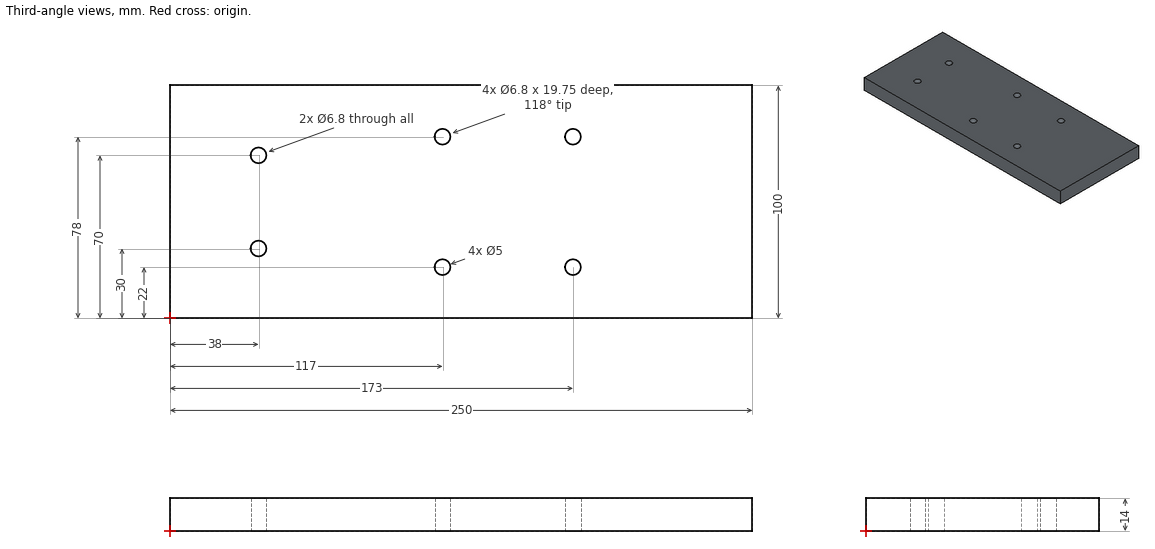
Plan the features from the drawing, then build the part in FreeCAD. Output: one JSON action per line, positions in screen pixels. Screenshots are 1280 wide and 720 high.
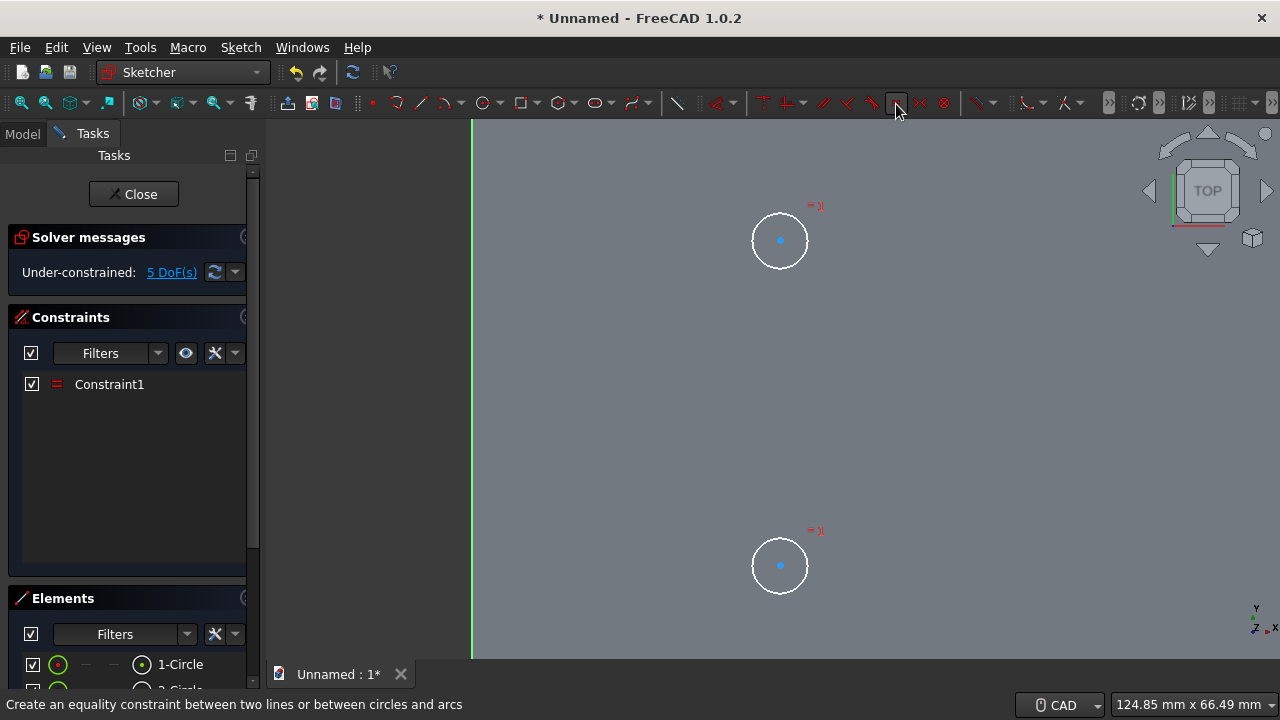
{"action": "left_click", "coordinate": [716, 104]}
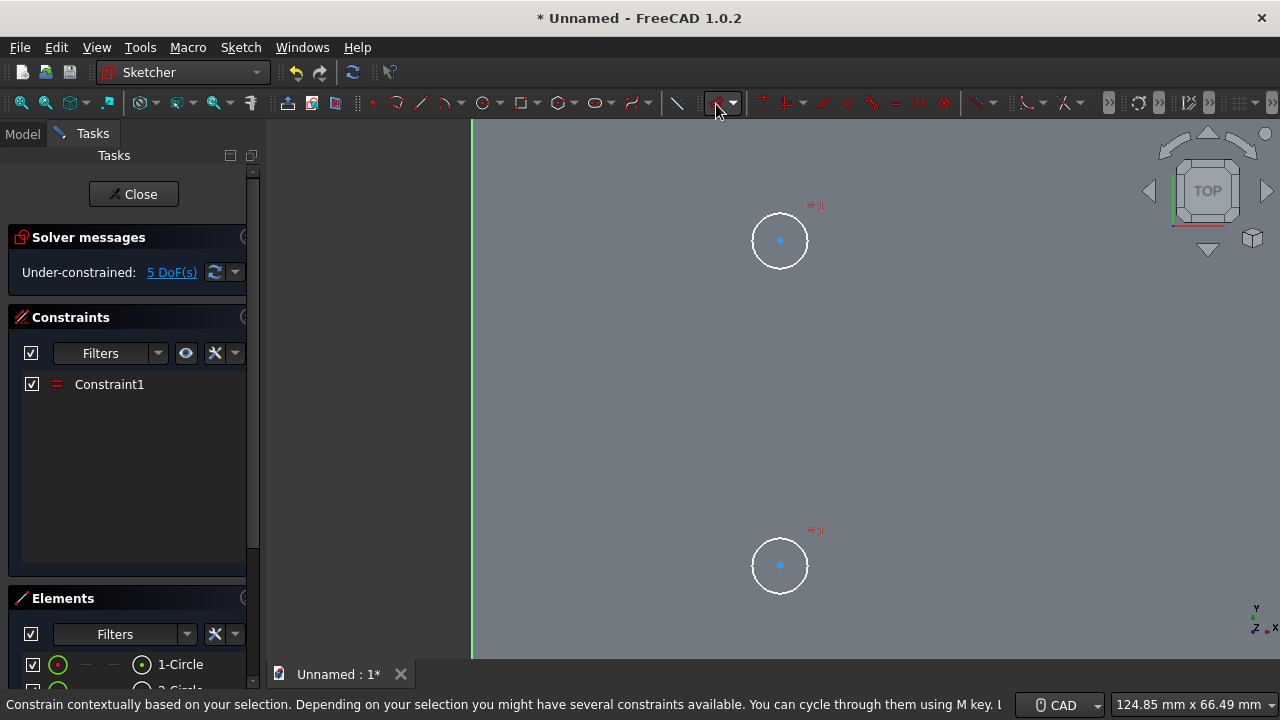
{"action": "left_click", "coordinate": [799, 221]}
{"action": "left_click", "coordinate": [821, 198]}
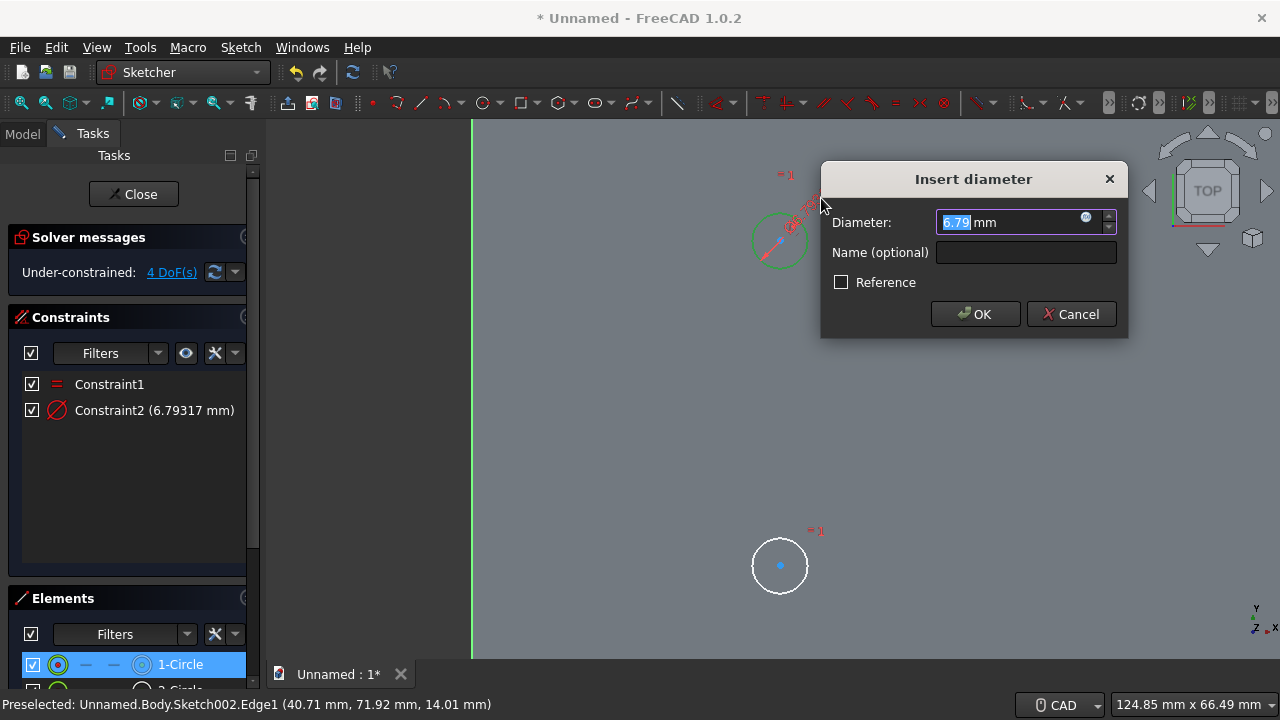
{"action": "type", "text": "6.8"}
{"action": "key", "text": "Return"}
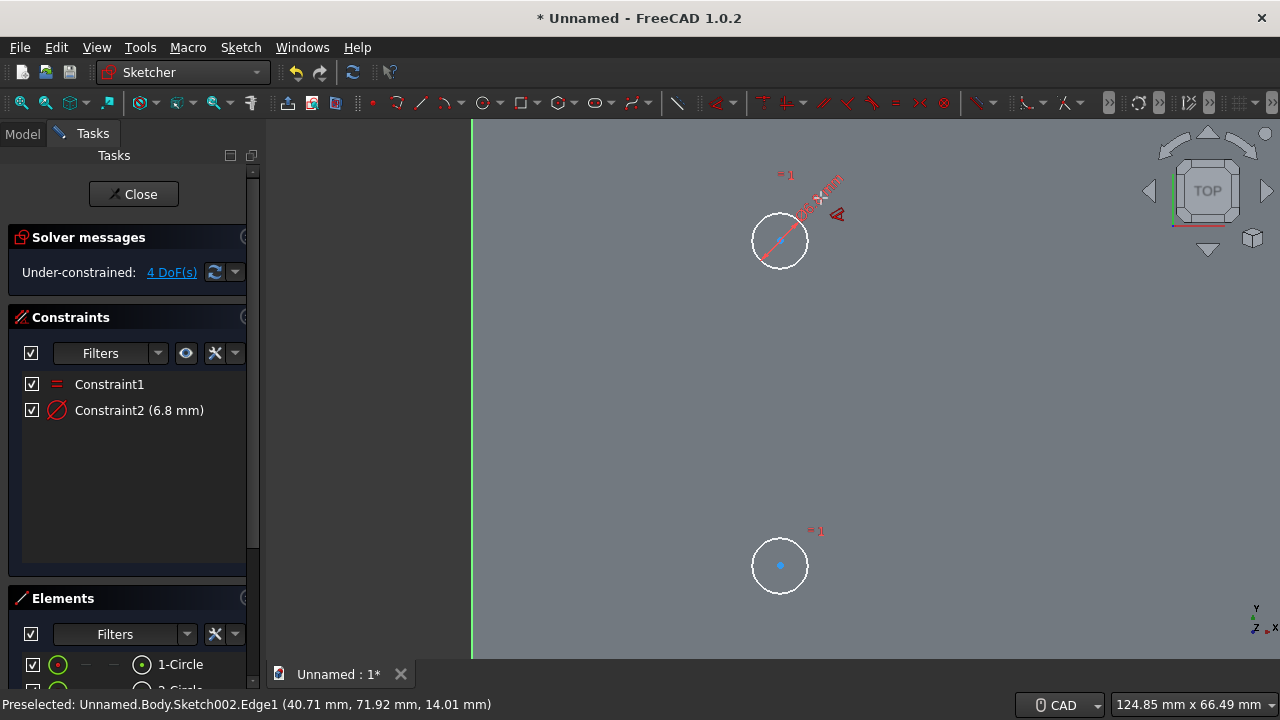
{"action": "left_click", "coordinate": [780, 241]}
{"action": "left_click", "coordinate": [626, 207]}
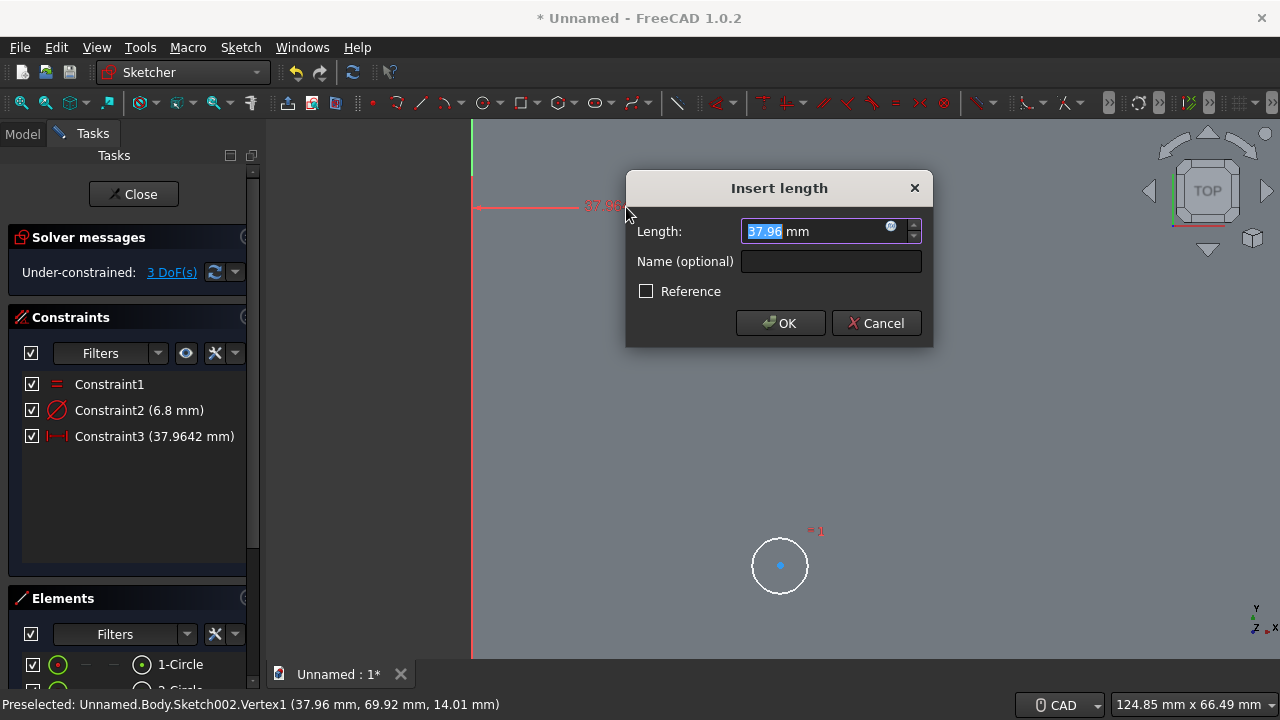
{"action": "type", "text": "38"}
{"action": "key", "text": "Return"}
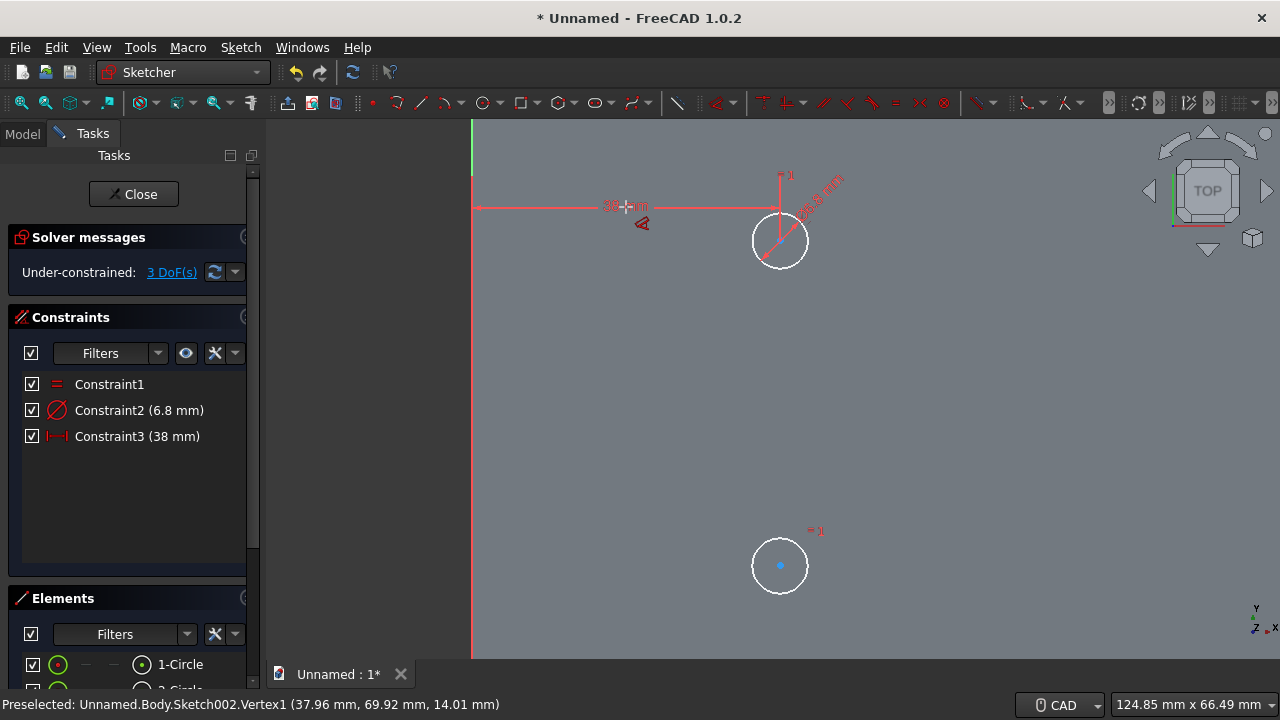
{"action": "left_click", "coordinate": [780, 241]}
{"action": "left_click", "coordinate": [438, 436]}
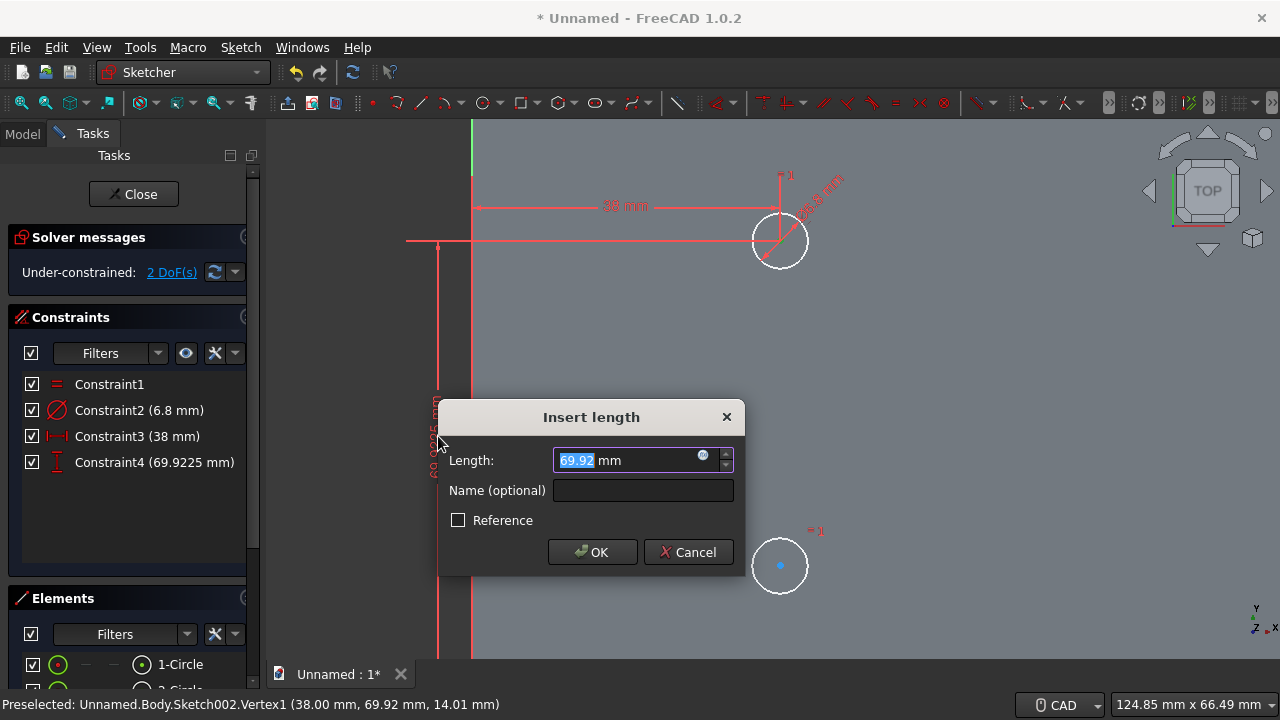
{"action": "type", "text": "70"}
{"action": "key", "text": "Return"}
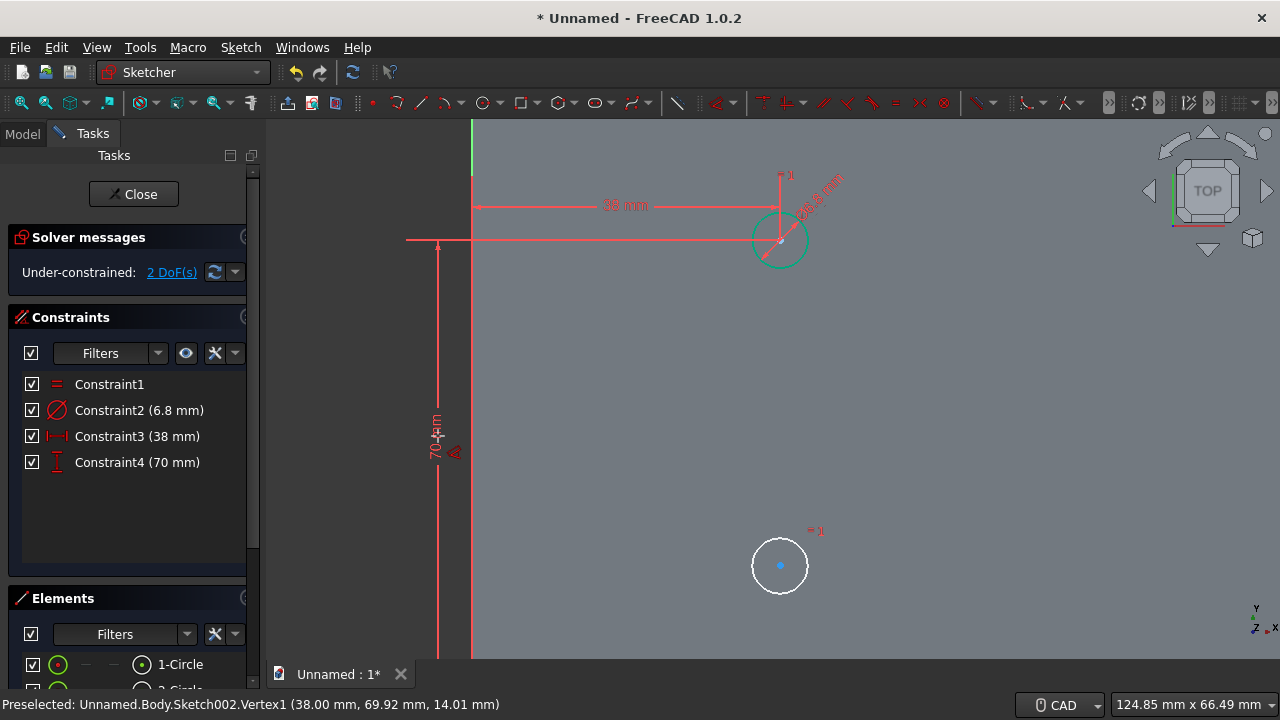
{"action": "left_click", "coordinate": [780, 566]}
{"action": "left_click", "coordinate": [626, 532]}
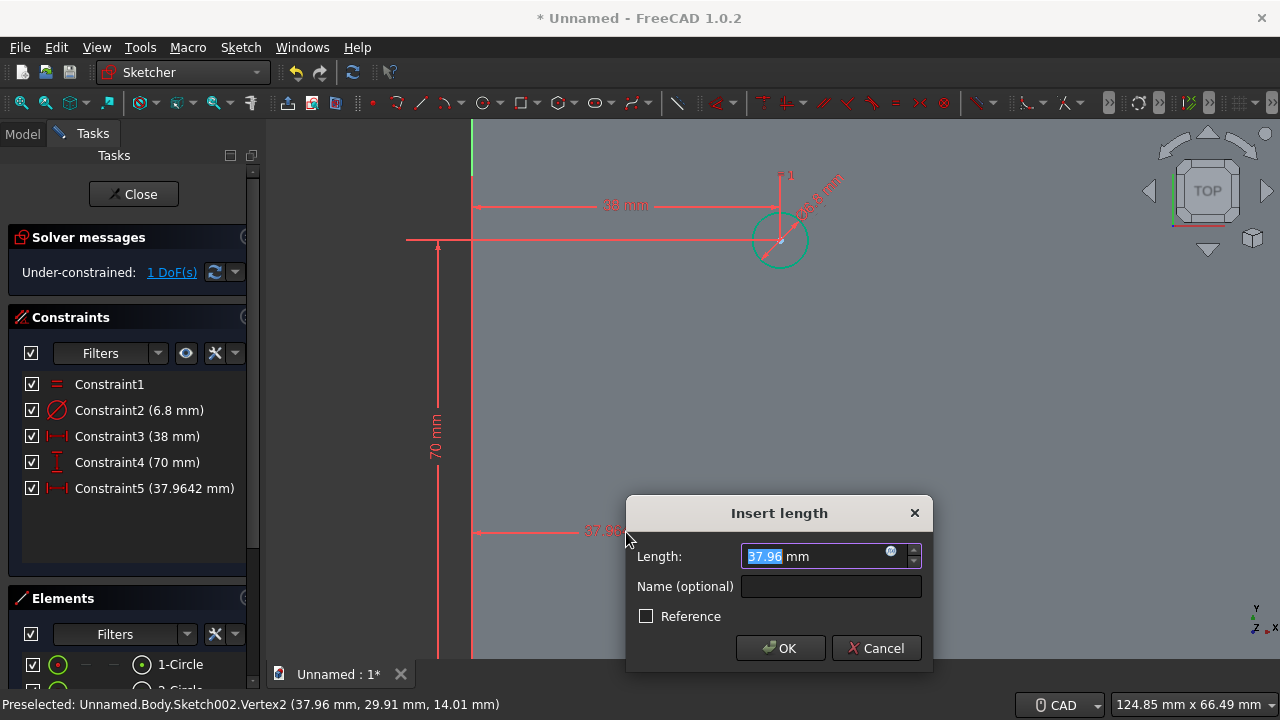
{"action": "type", "text": "38"}
{"action": "key", "text": "Return"}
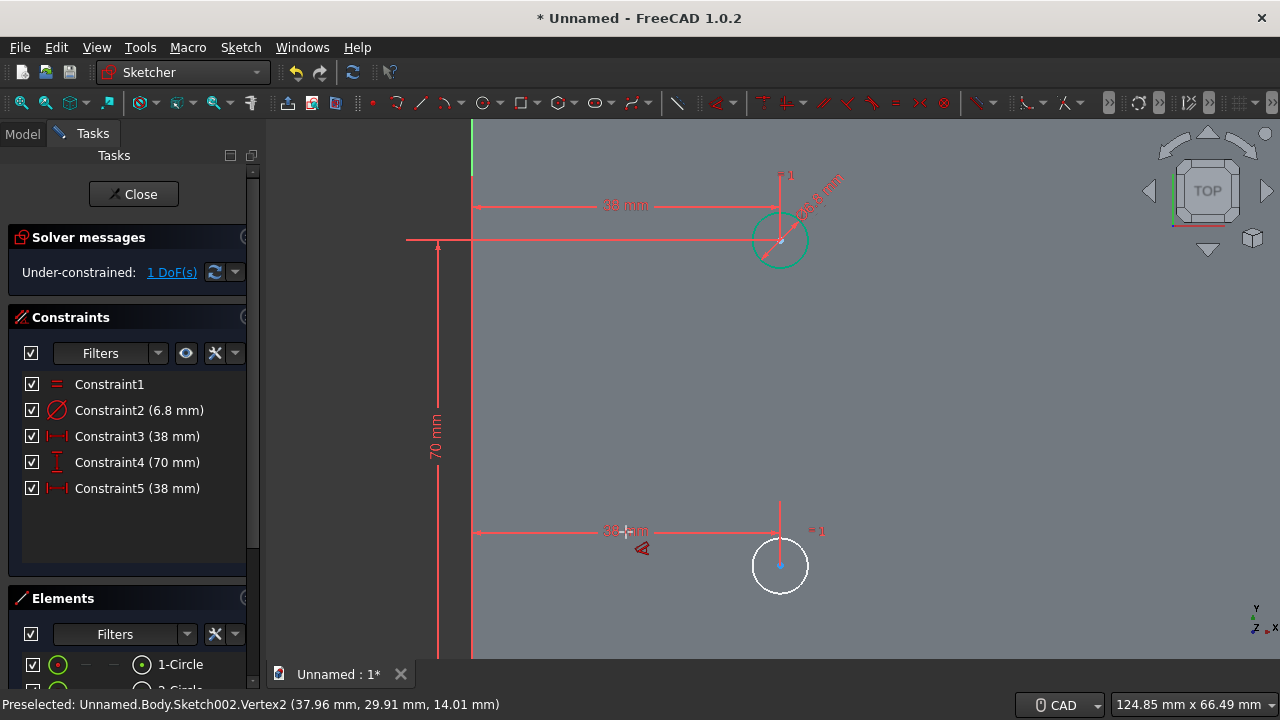
{"action": "left_click", "coordinate": [780, 566]}
{"action": "left_click", "coordinate": [438, 598]}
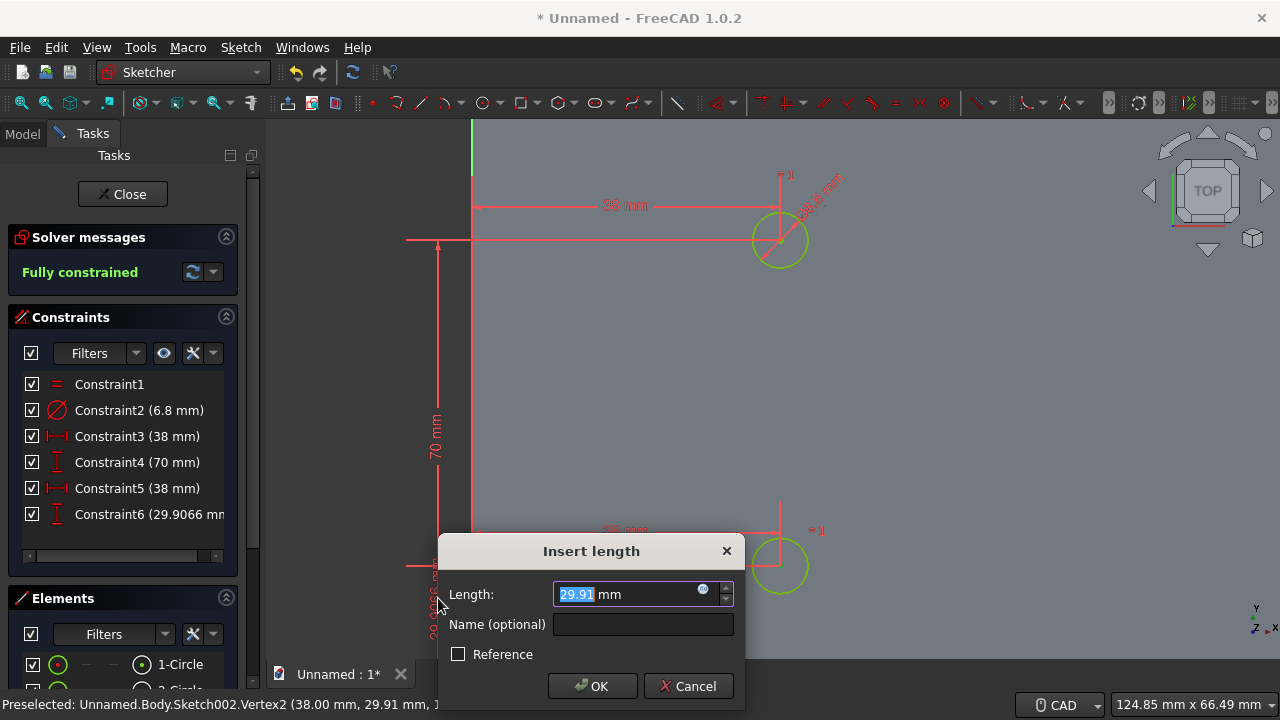
{"action": "type", "text": "30"}
{"action": "key", "text": "Return"}
{"action": "key", "text": "Escape"}